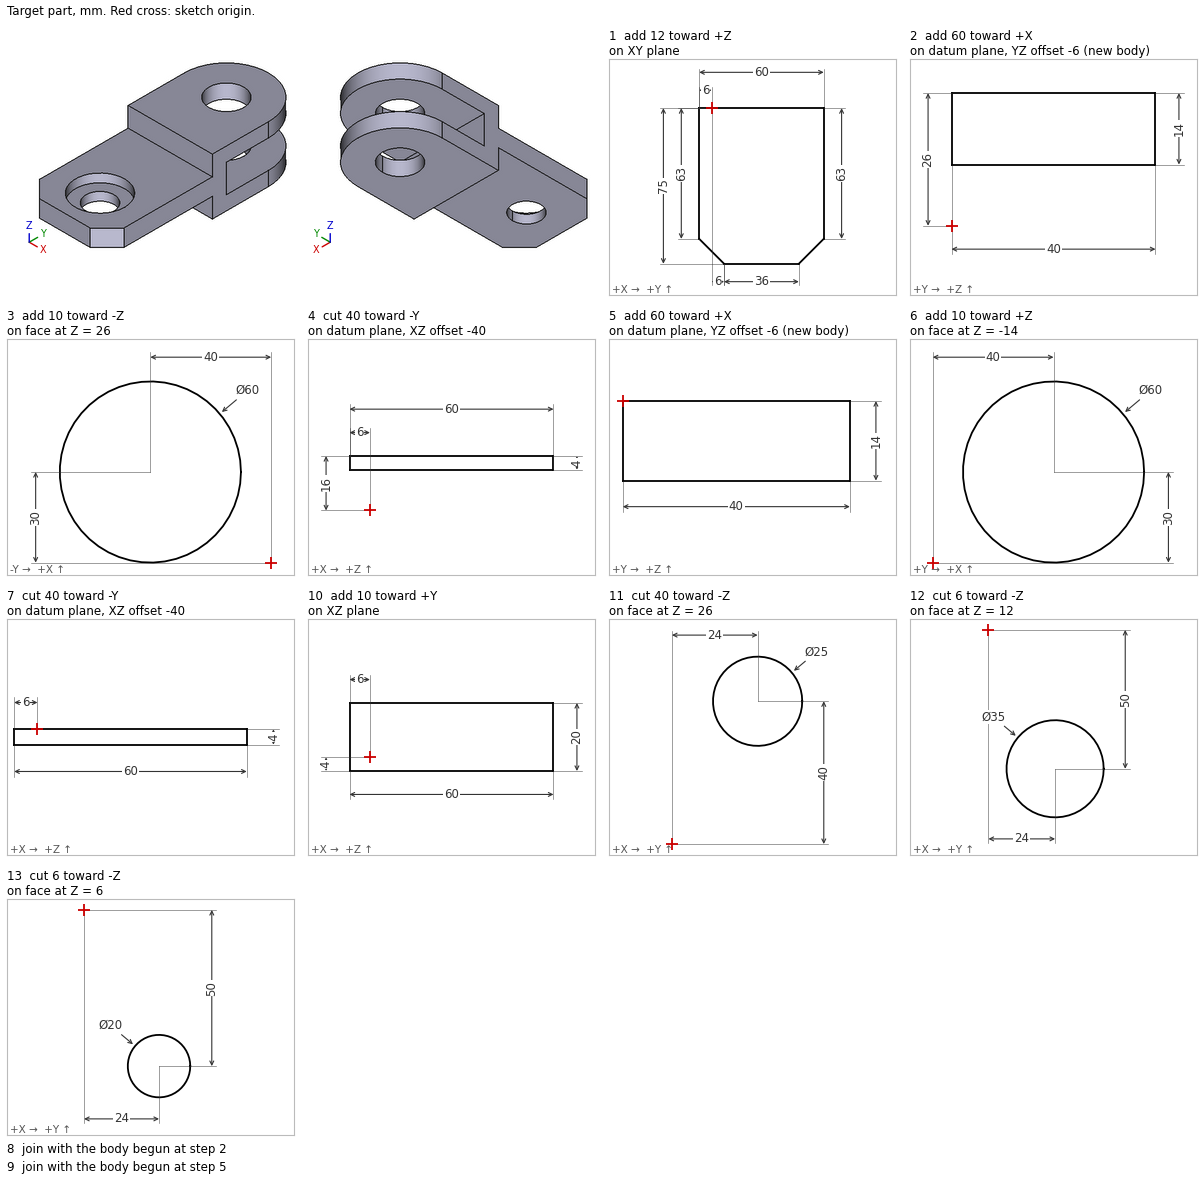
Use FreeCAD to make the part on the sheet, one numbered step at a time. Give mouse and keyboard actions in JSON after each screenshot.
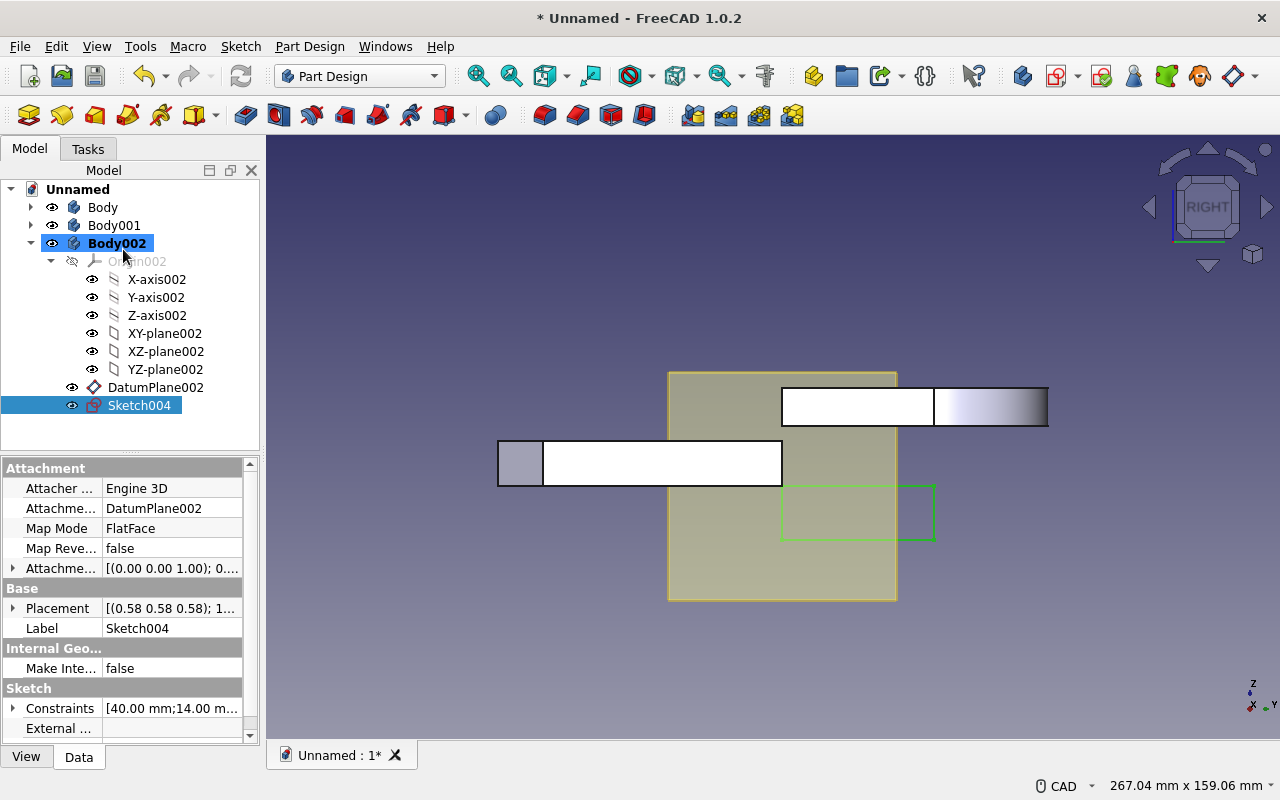
{"action": "left_click", "coordinate": [29, 116]}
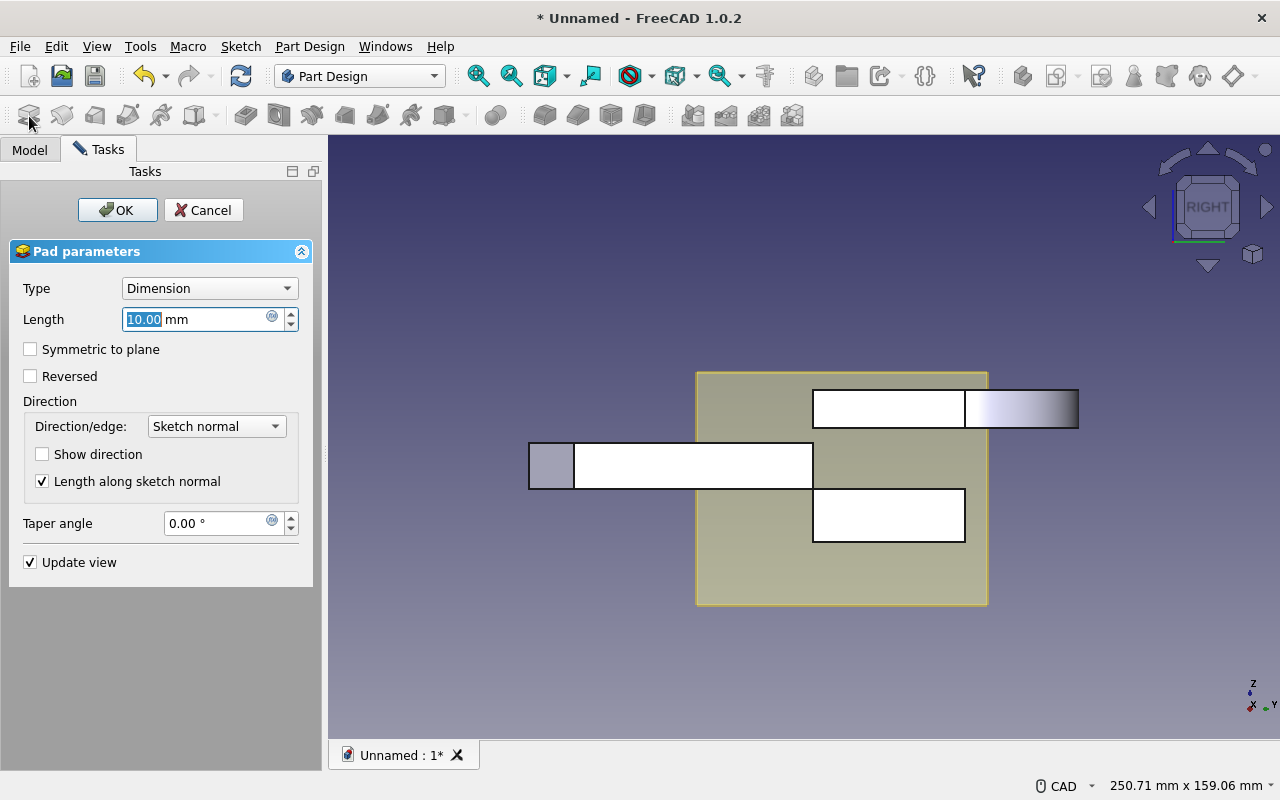
{"action": "type", "text": "60"}
{"action": "key", "text": "Tab"}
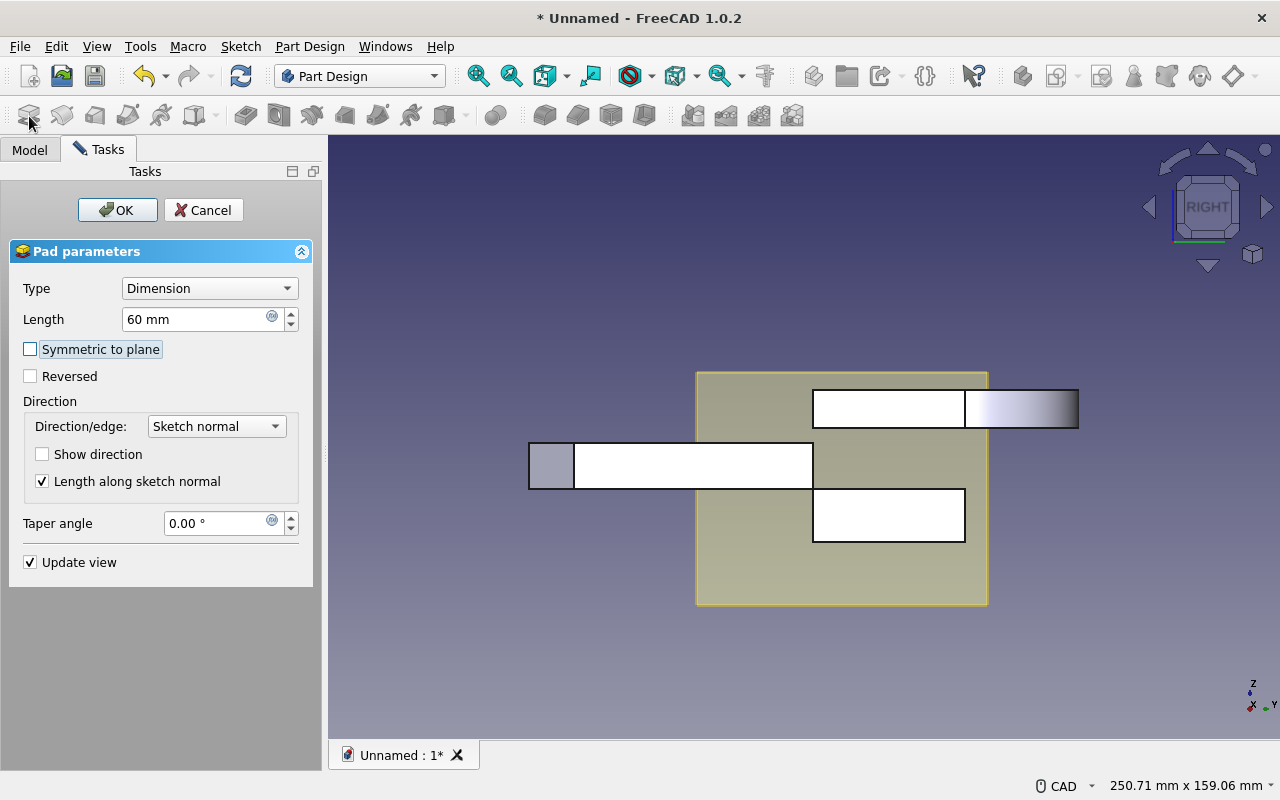
{"action": "left_click", "coordinate": [118, 210]}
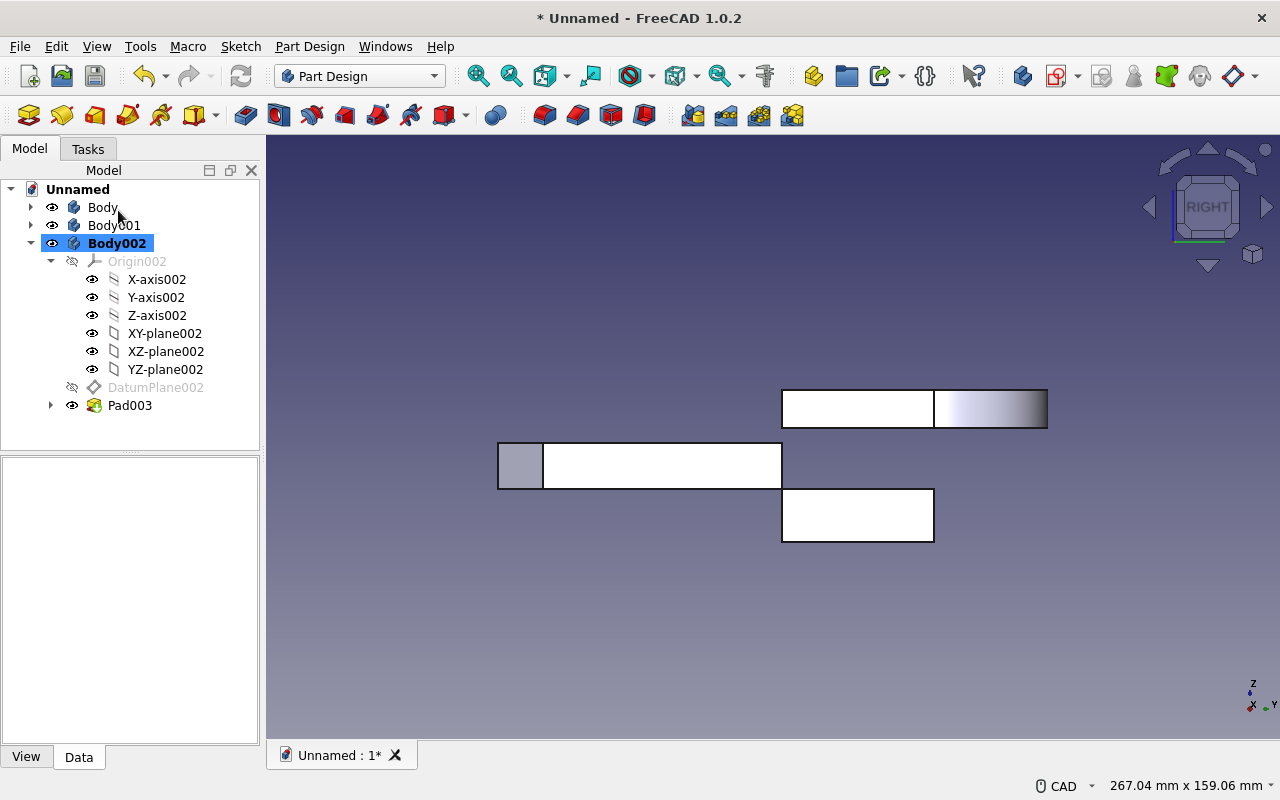
{"action": "left_click", "coordinate": [479, 76]}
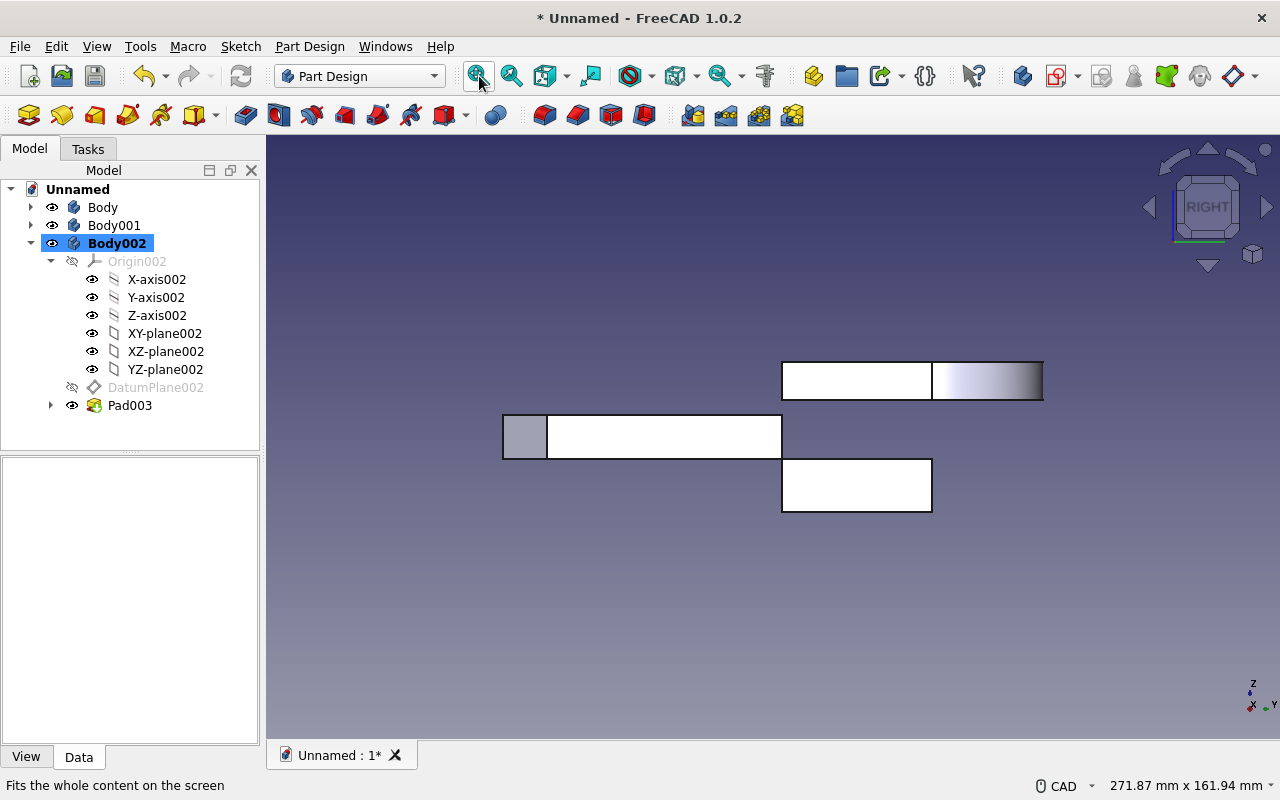
{"action": "key", "text": "5"}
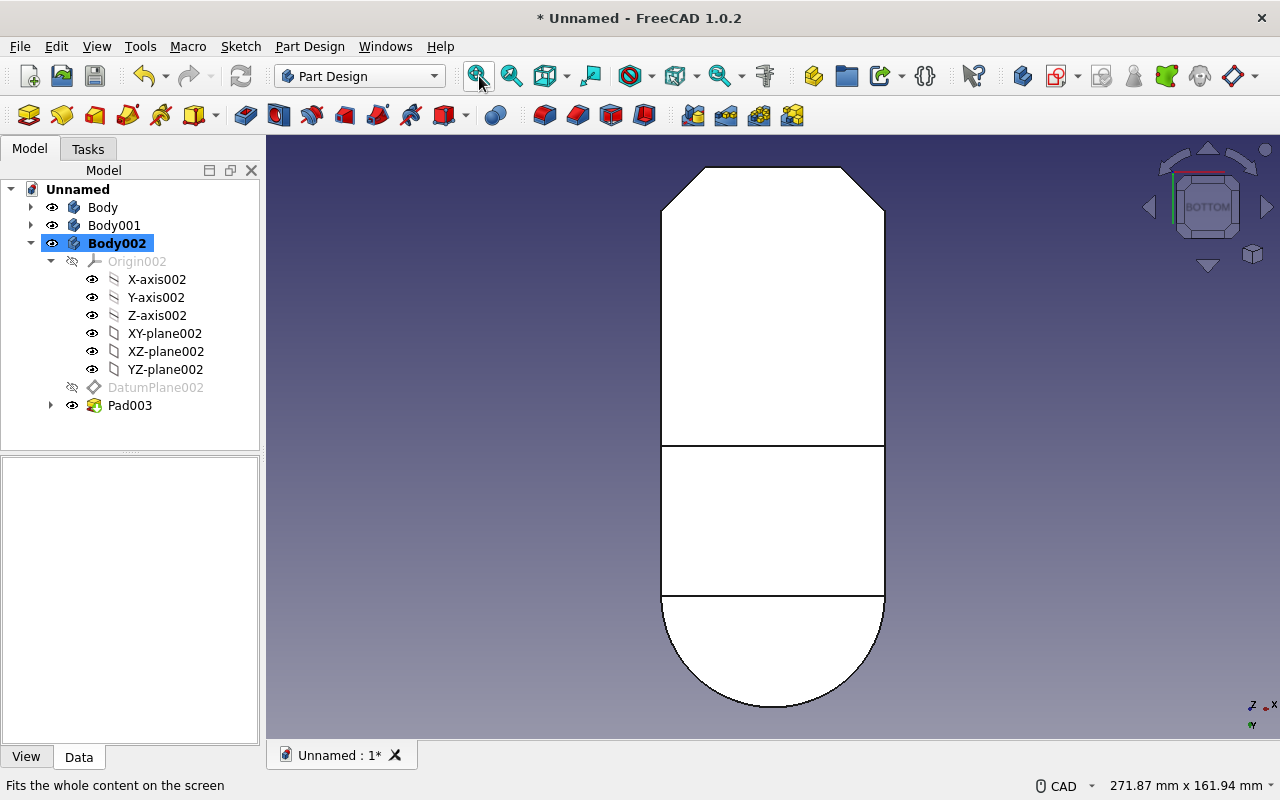
{"action": "left_click", "coordinate": [479, 76]}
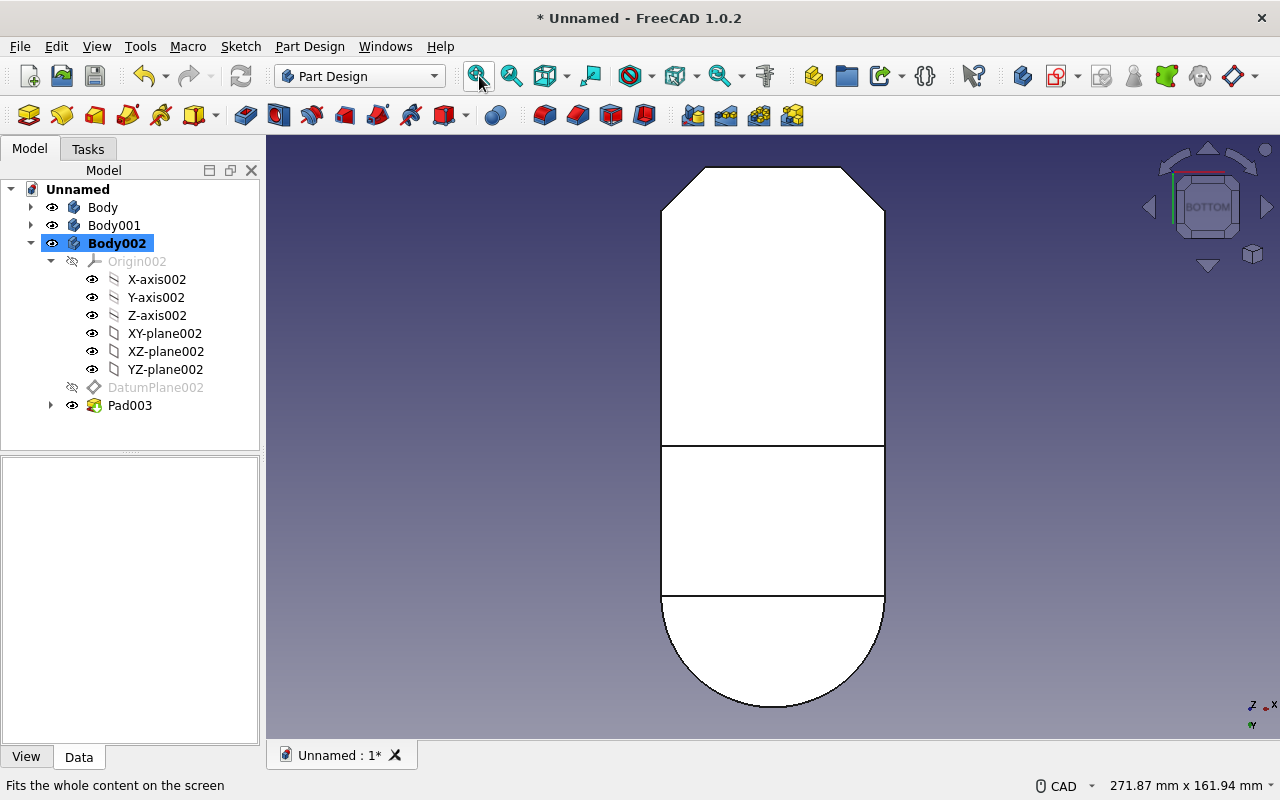
{"action": "left_click", "coordinate": [805, 520]}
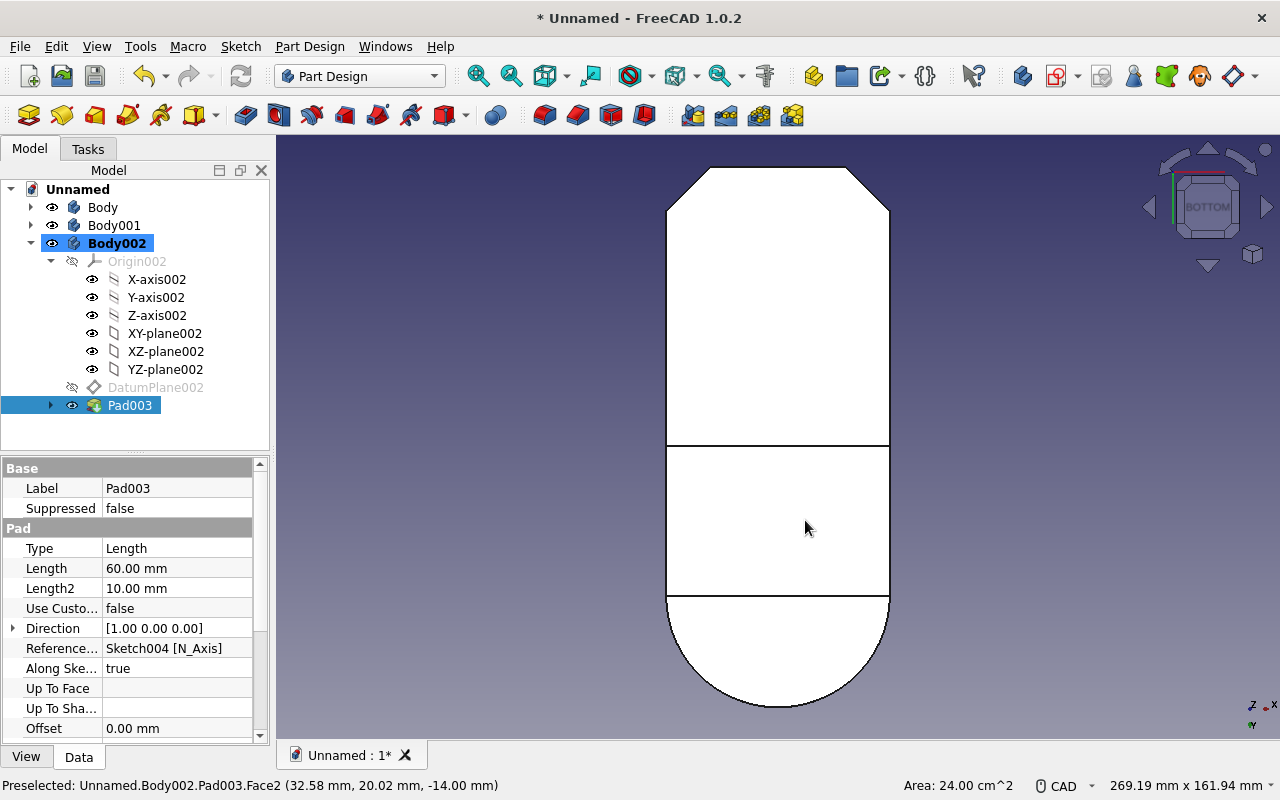
{"action": "left_click", "coordinate": [1056, 76]}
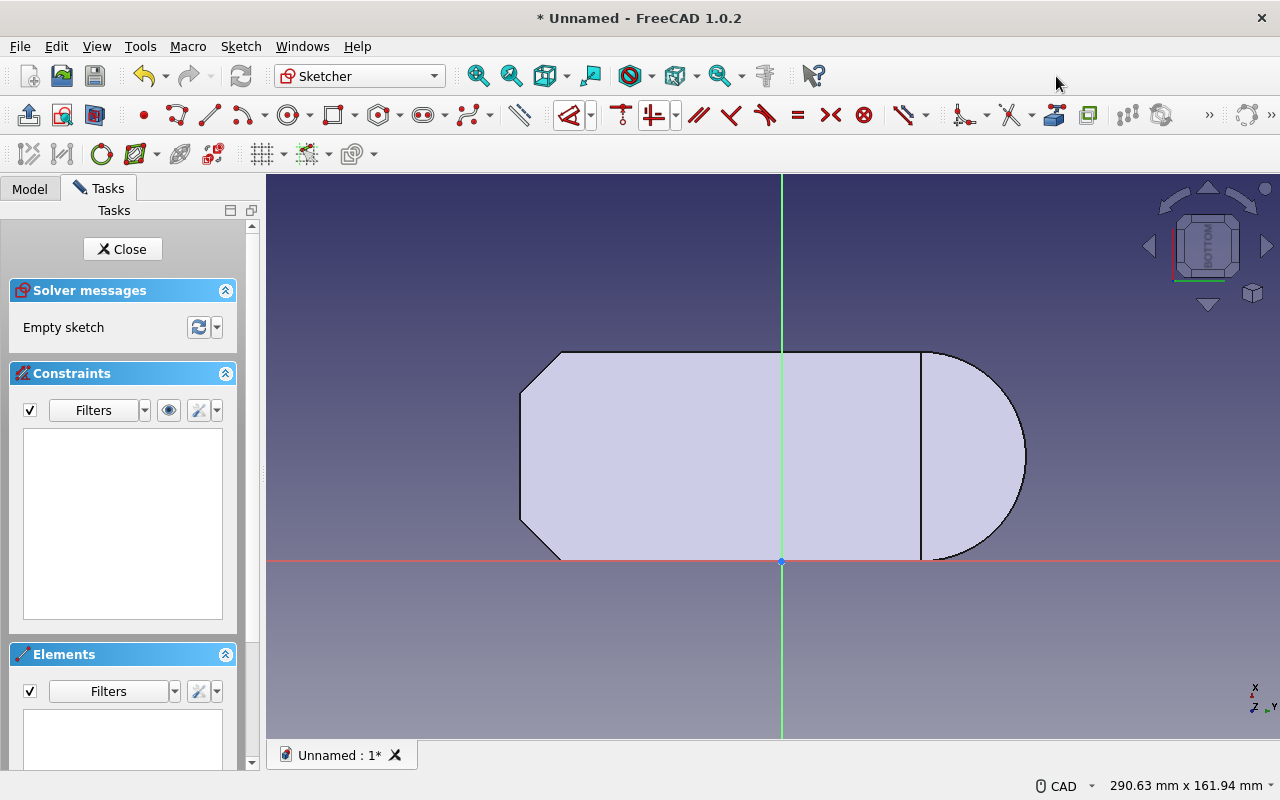
{"action": "scroll", "coordinate": [1115, 456], "scroll_direction": "up", "scroll_amount": 3}